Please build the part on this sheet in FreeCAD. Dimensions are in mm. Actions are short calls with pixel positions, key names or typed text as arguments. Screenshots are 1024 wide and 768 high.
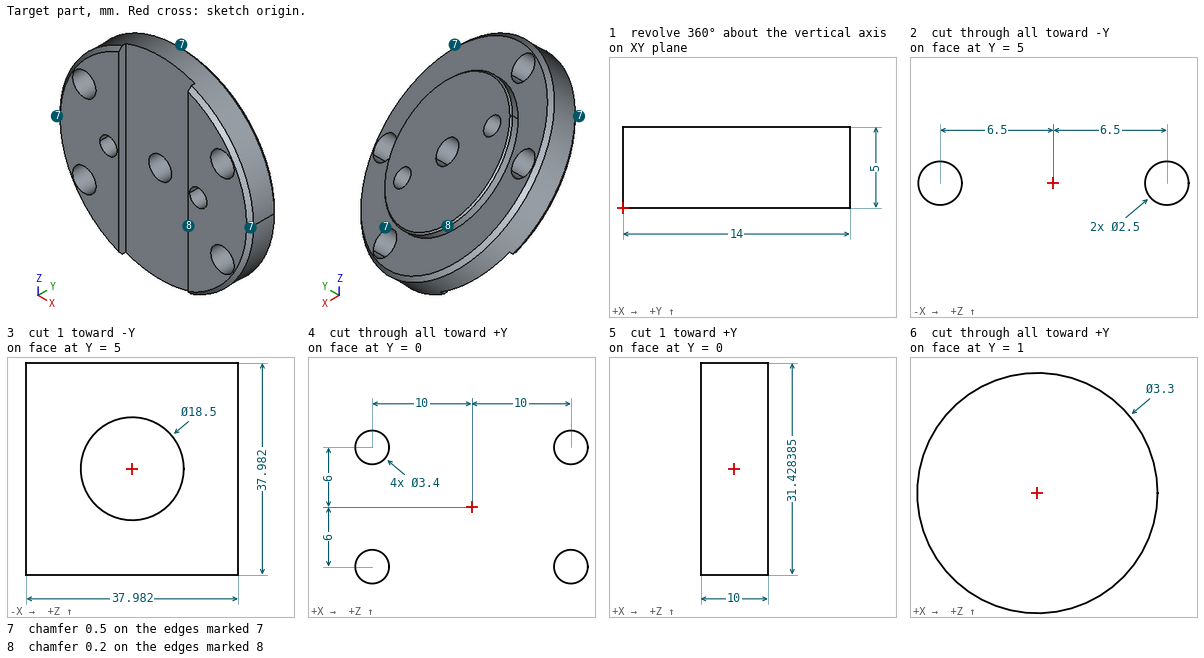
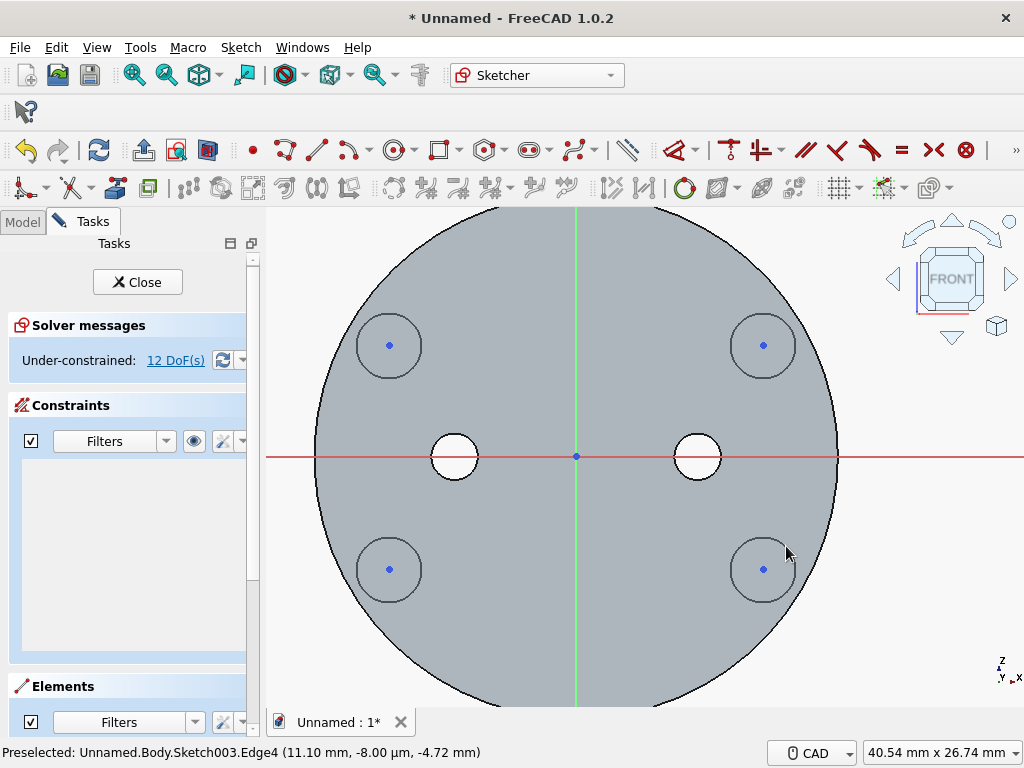
click(412, 323)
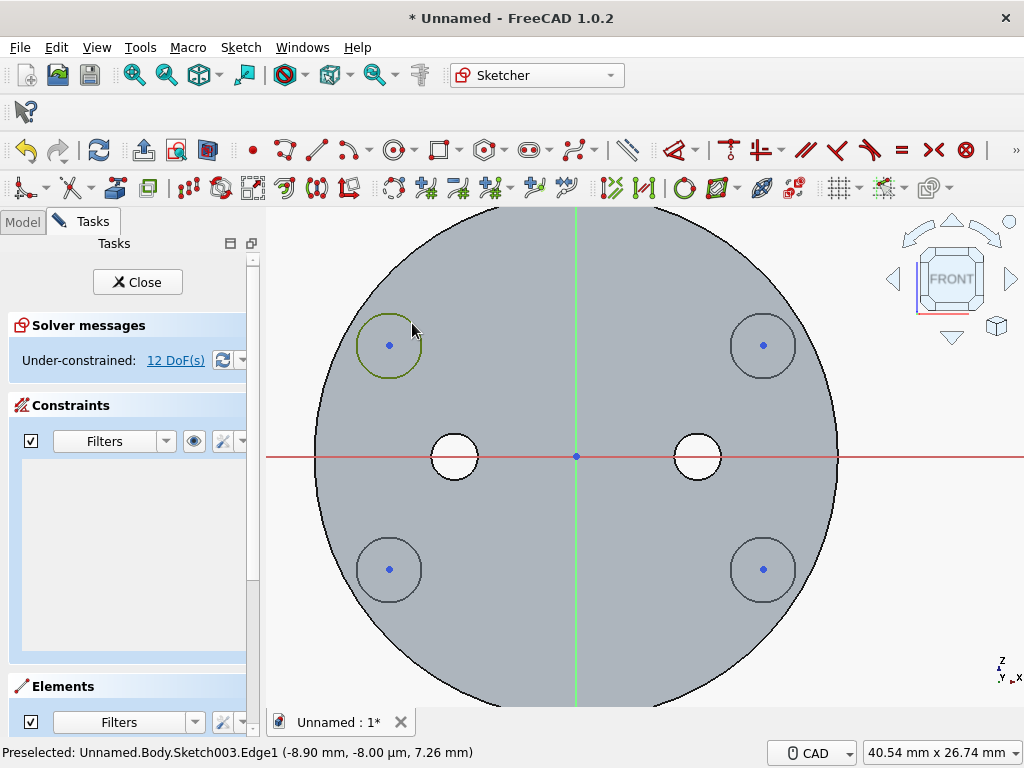
click(412, 547)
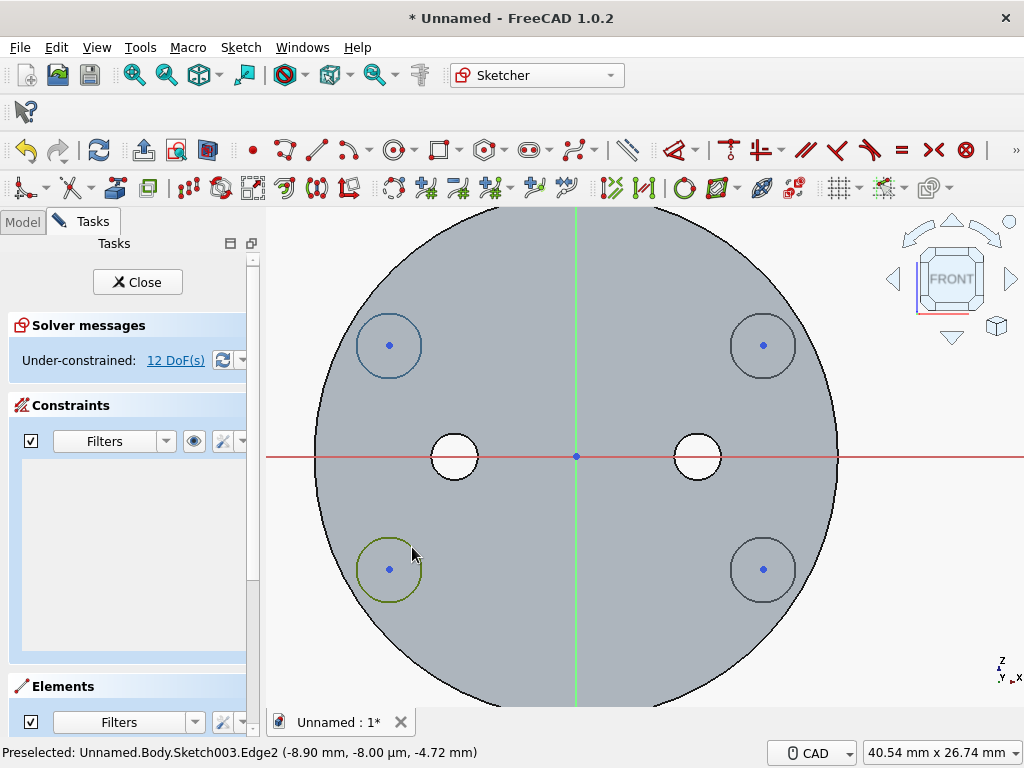
click(786, 323)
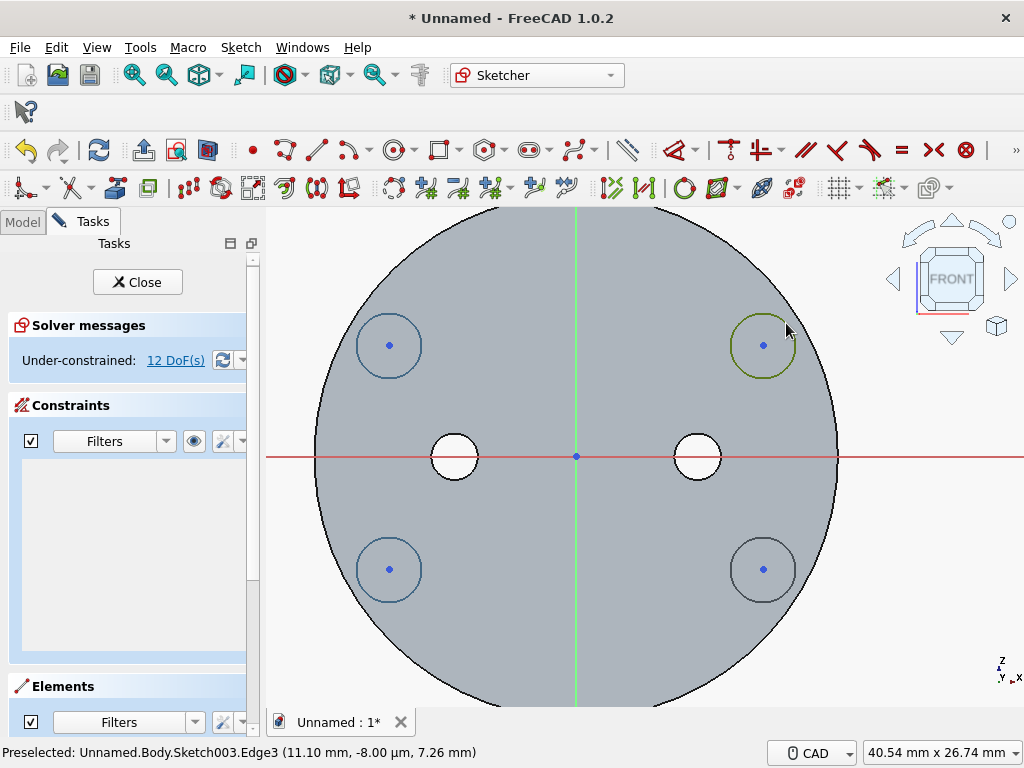
click(786, 547)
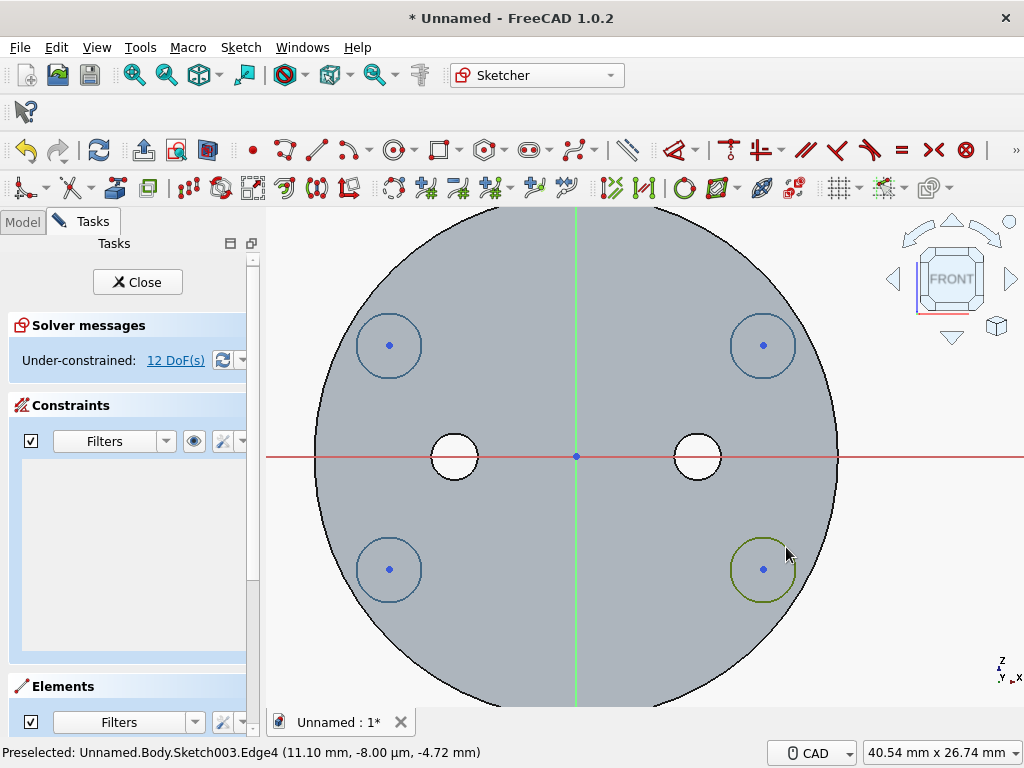
key(e)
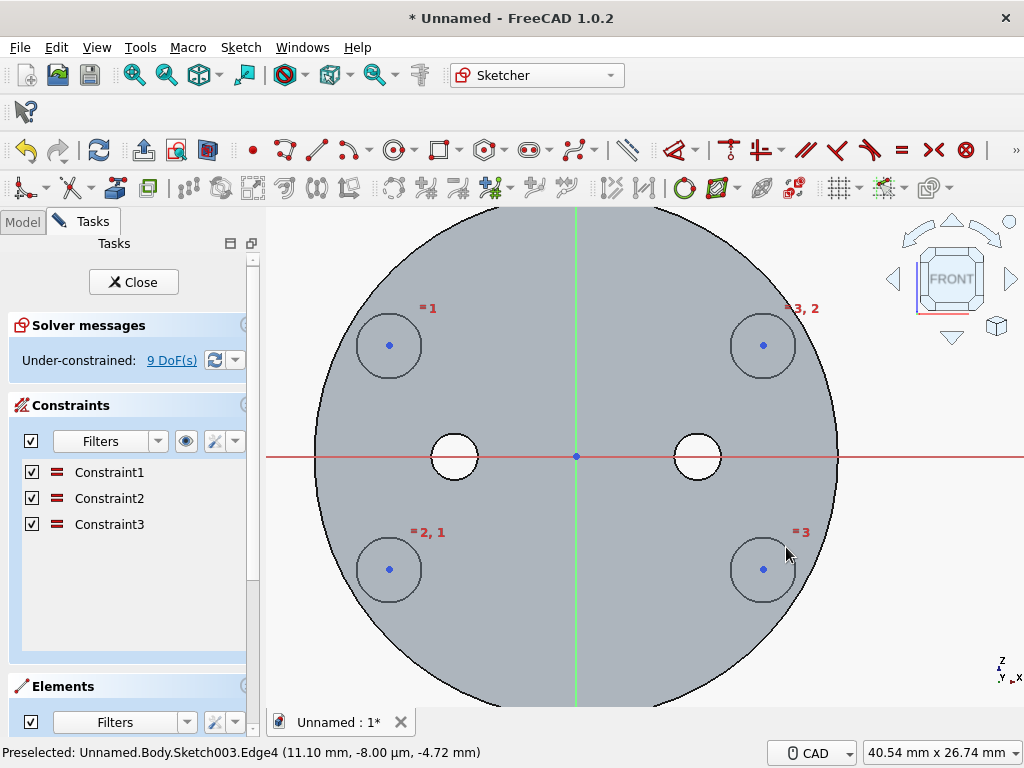
click(389, 346)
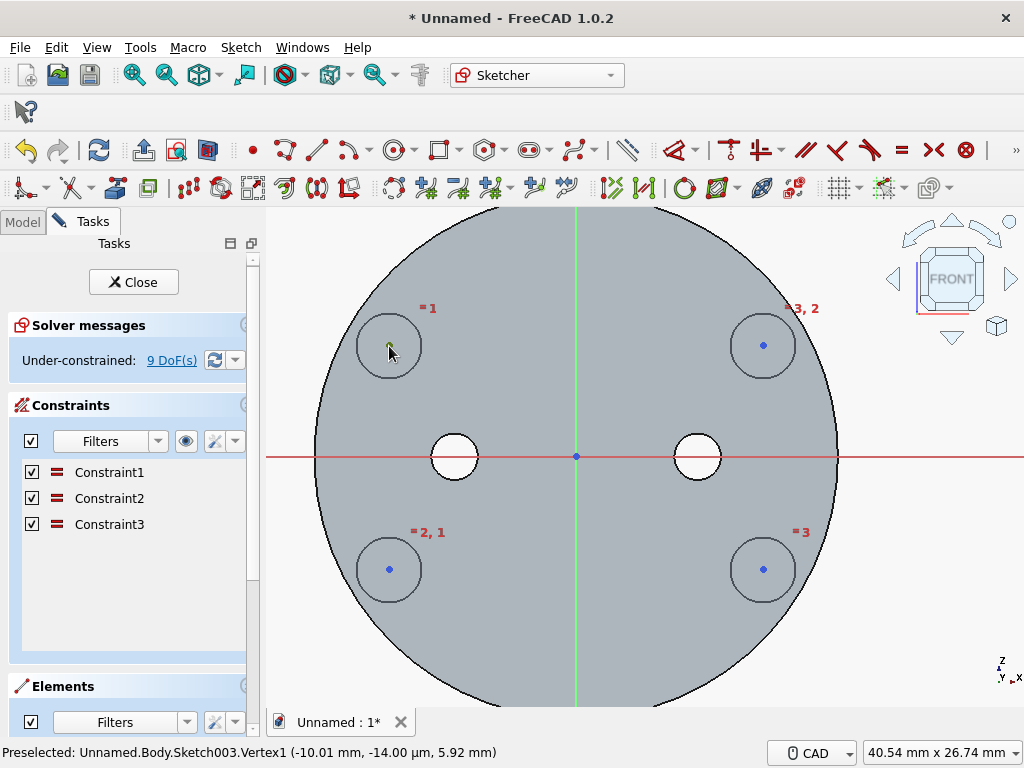
click(389, 570)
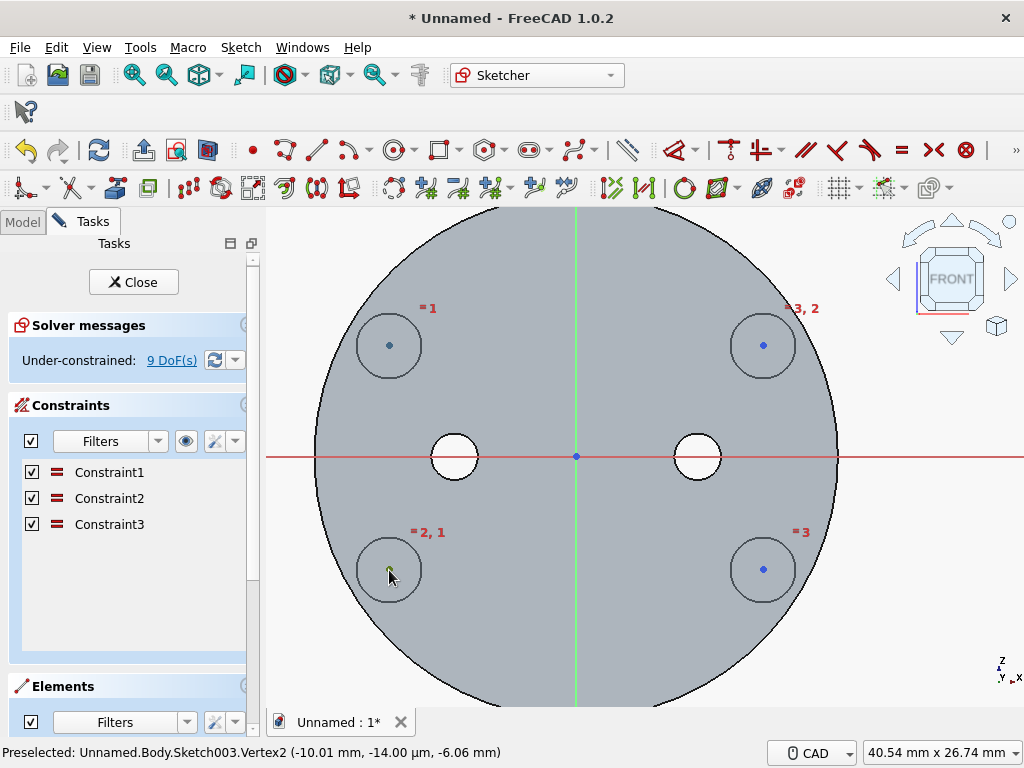
key(v)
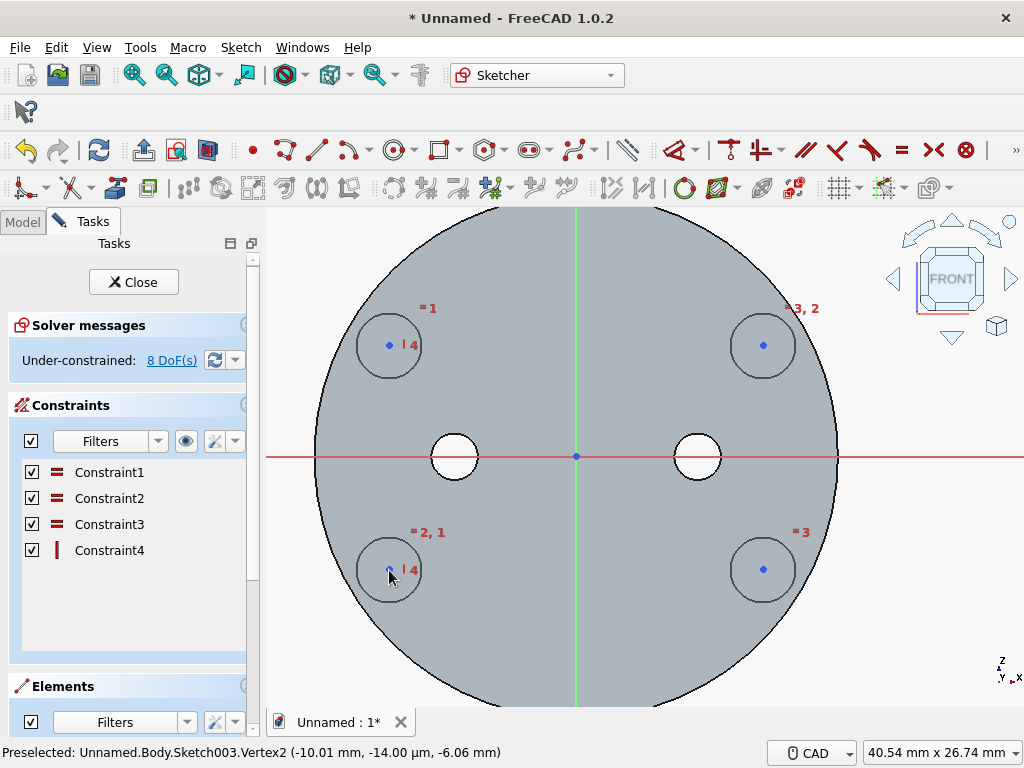
click(389, 346)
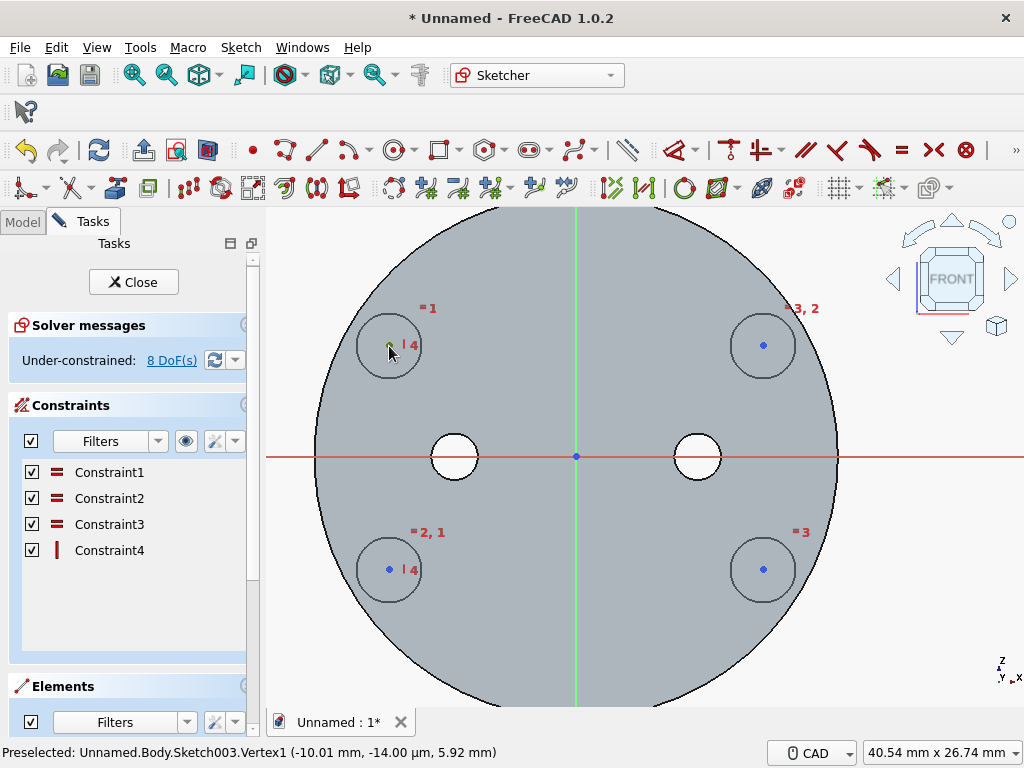
click(763, 346)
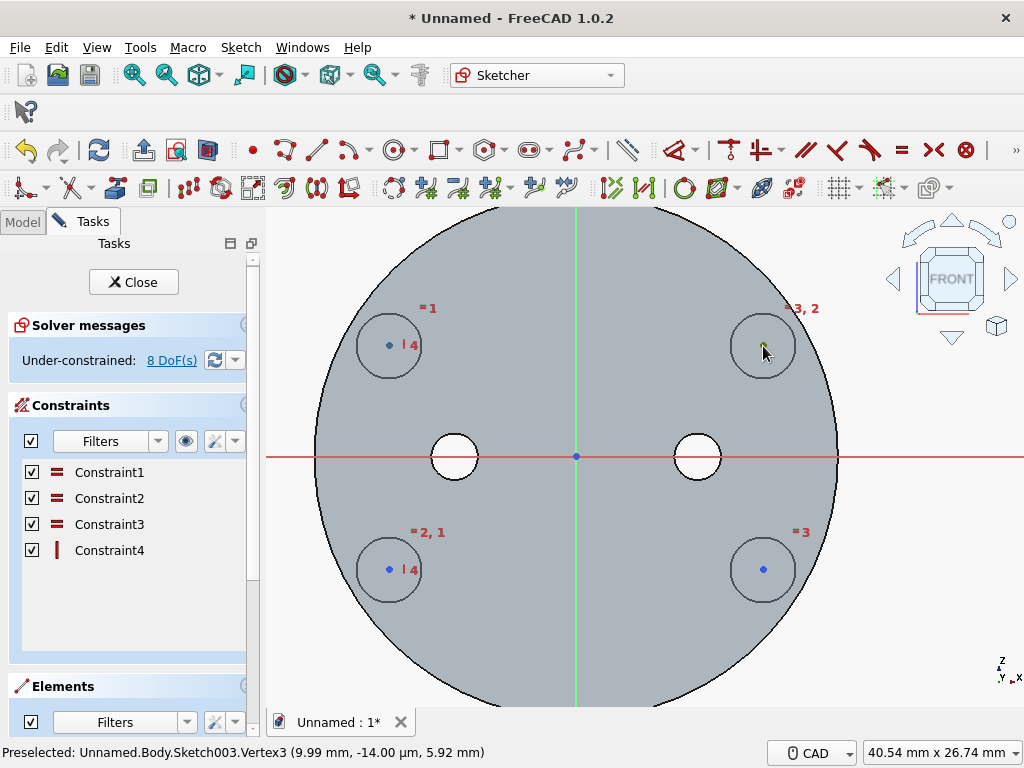
key(h)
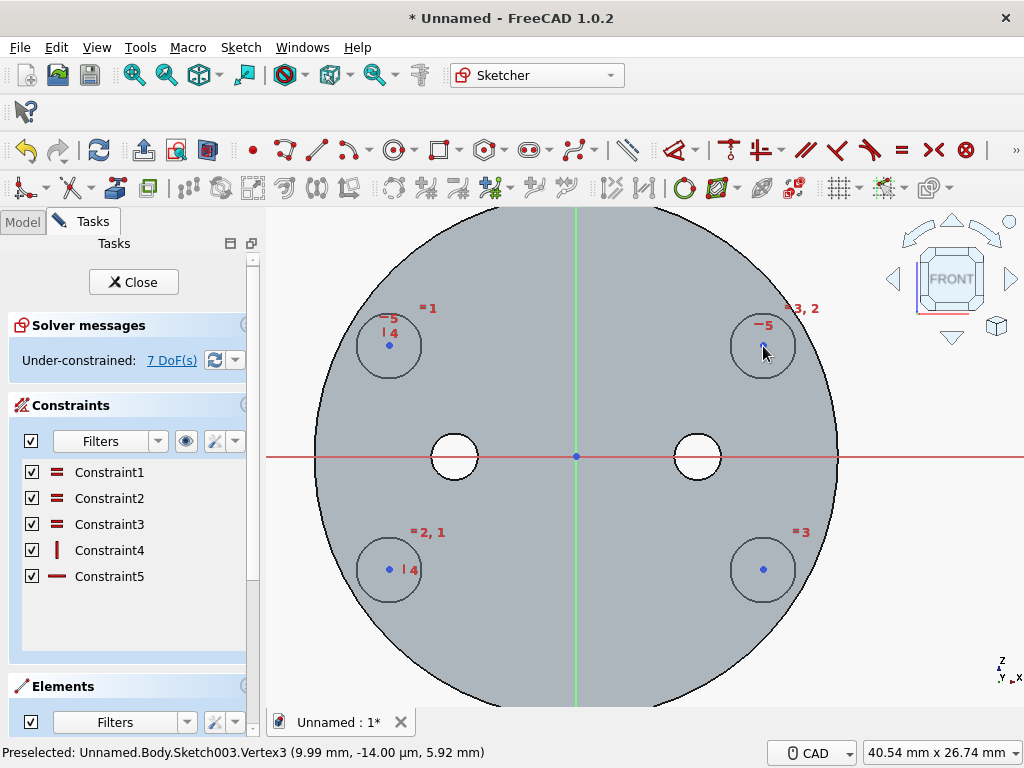
click(763, 346)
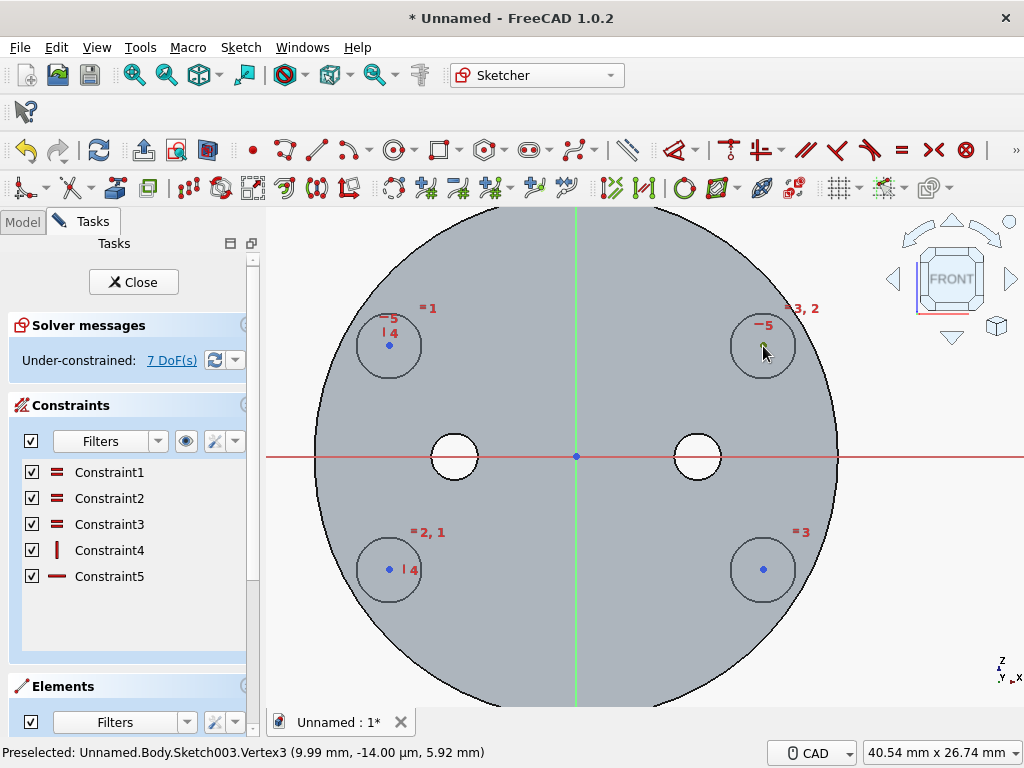
click(763, 570)